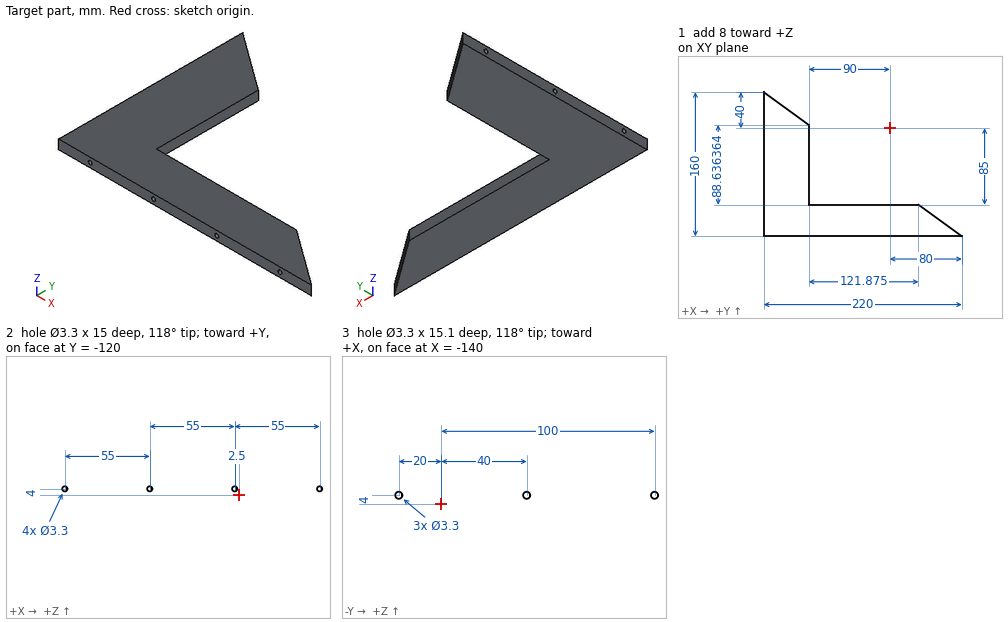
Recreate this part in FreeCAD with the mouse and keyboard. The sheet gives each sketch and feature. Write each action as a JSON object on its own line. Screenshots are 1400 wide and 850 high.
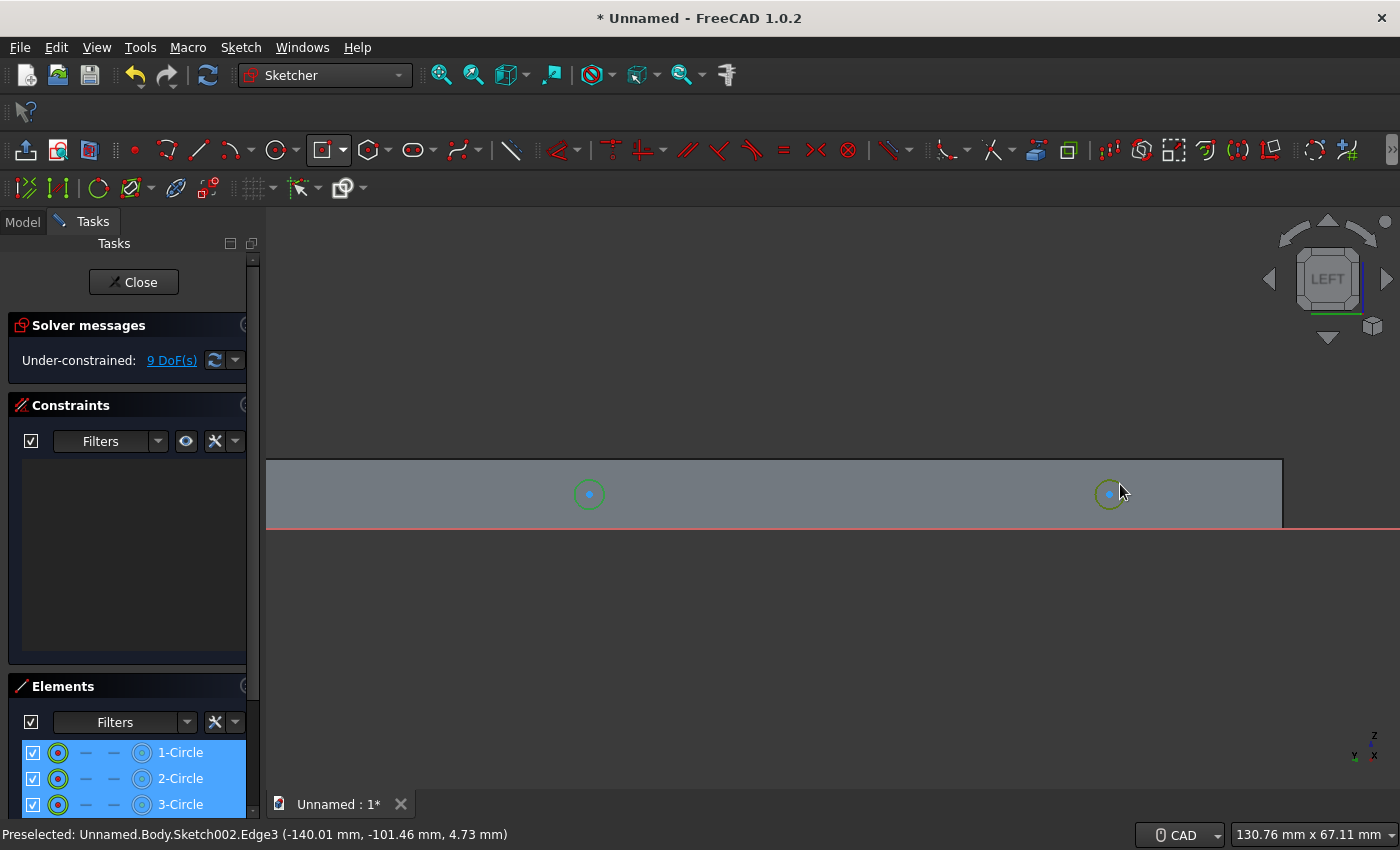
{"action": "key", "text": "e"}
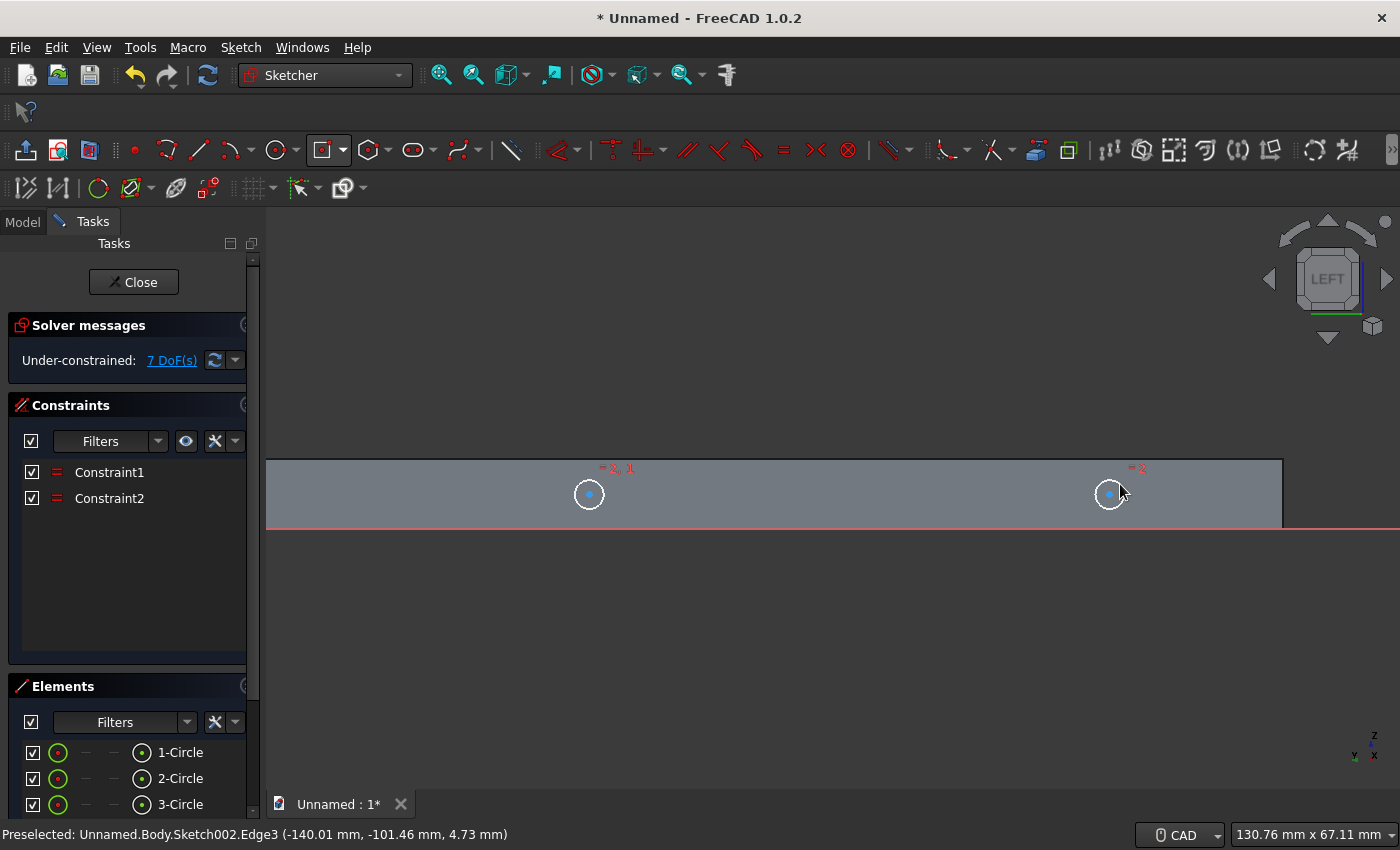
{"action": "scroll", "coordinate": [1120, 485], "scroll_direction": "down", "scroll_amount": 2}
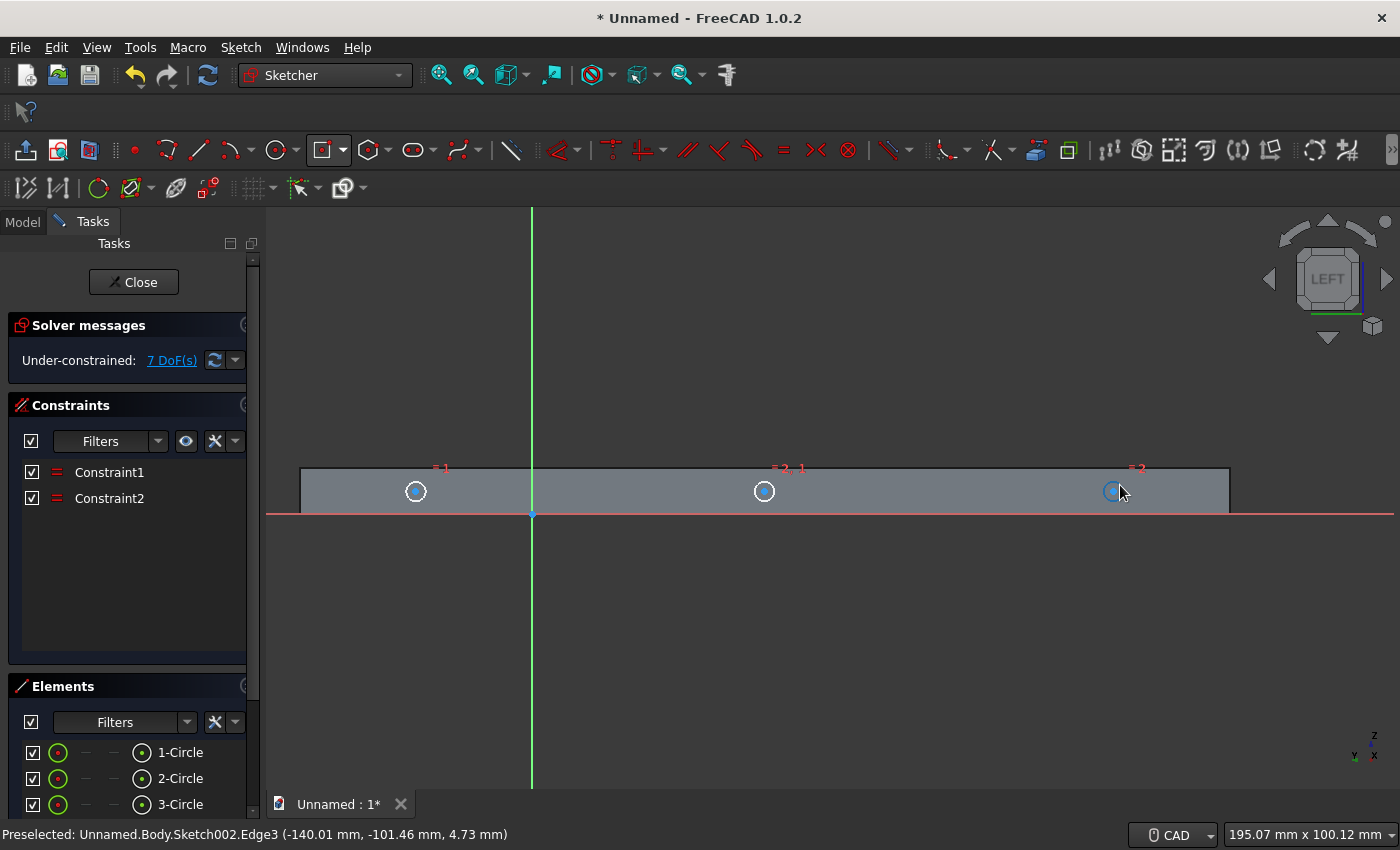
{"action": "left_click", "coordinate": [416, 492]}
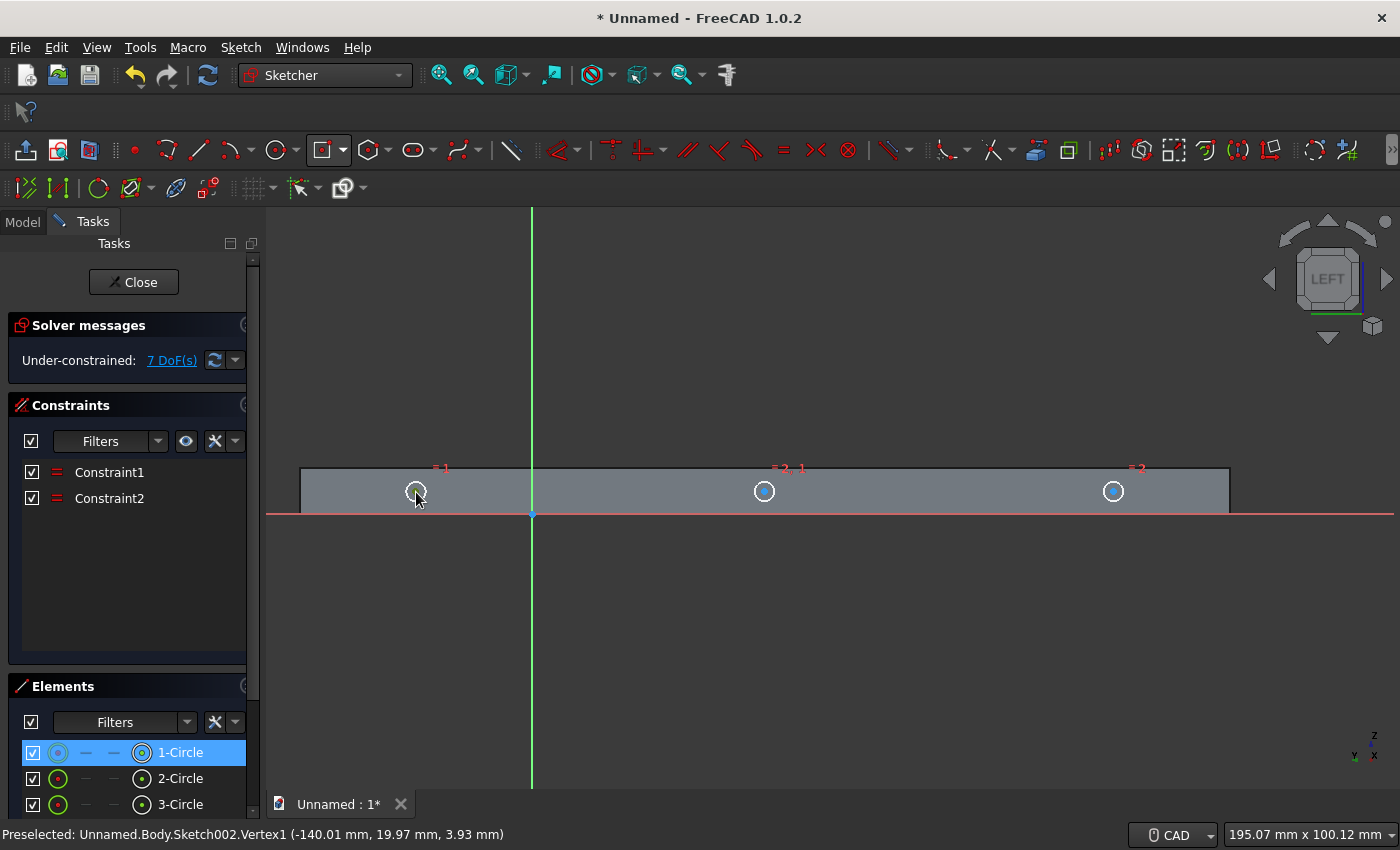
{"action": "left_click", "coordinate": [765, 492]}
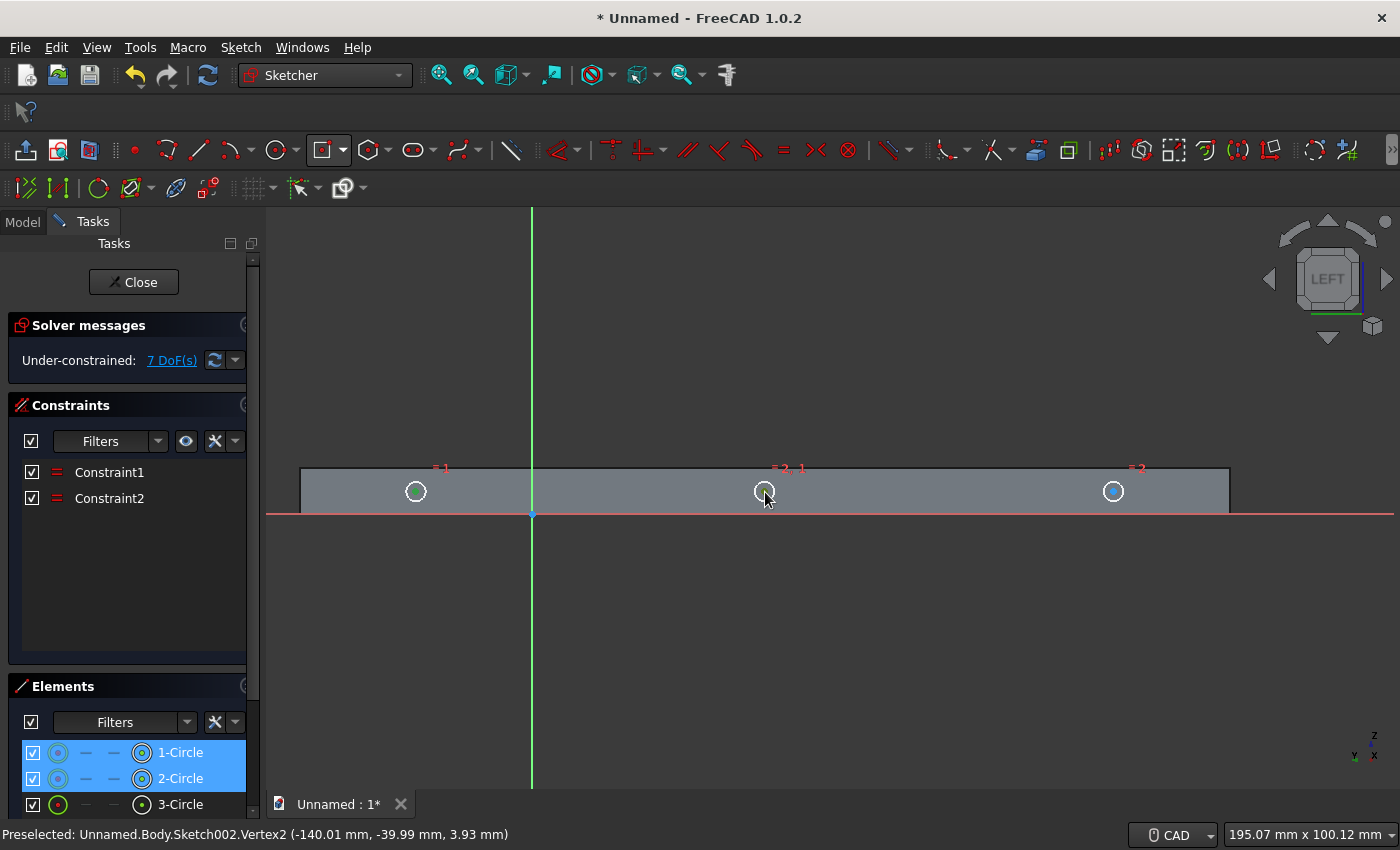
{"action": "left_click", "coordinate": [666, 150]}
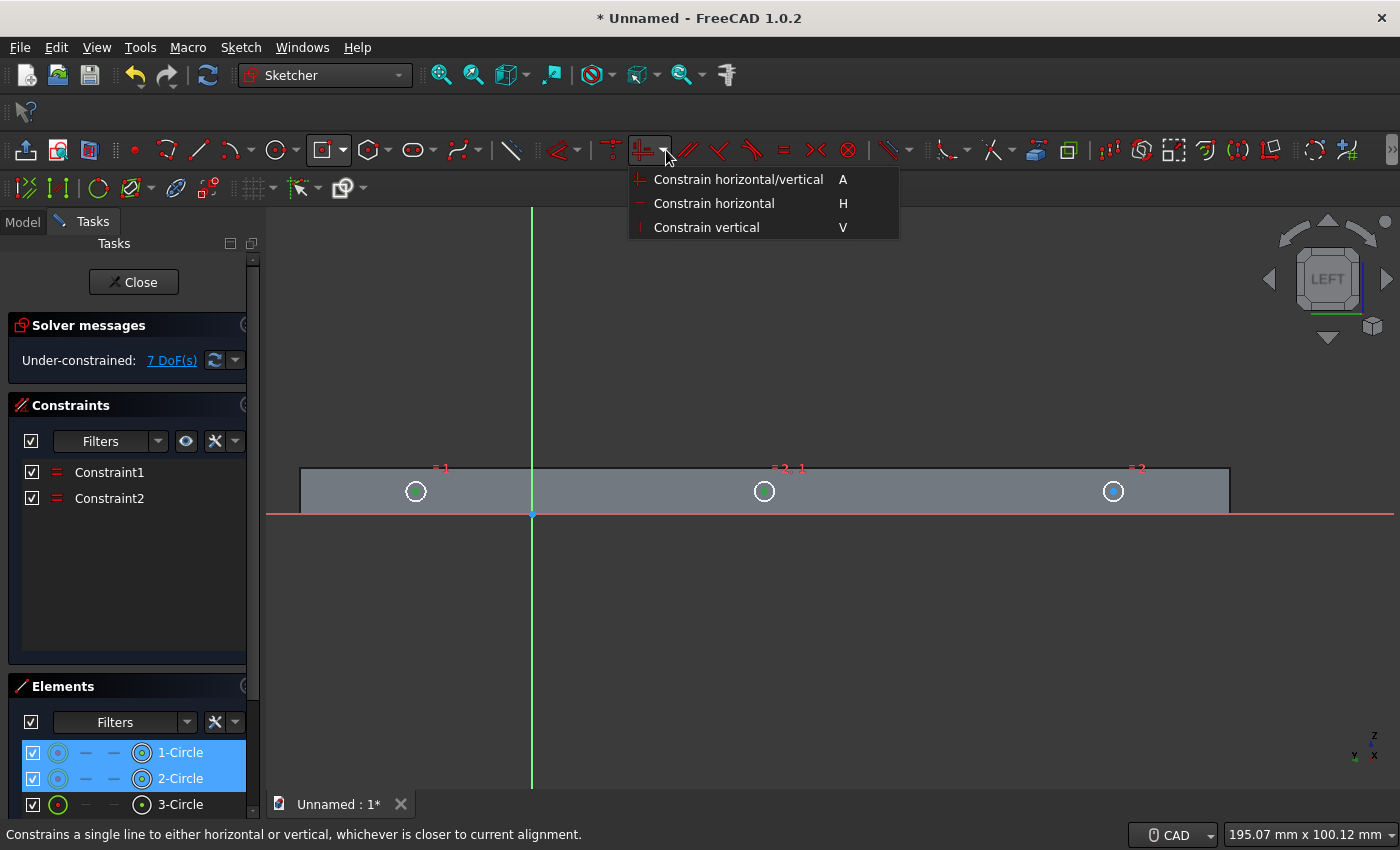
{"action": "left_click", "coordinate": [764, 203]}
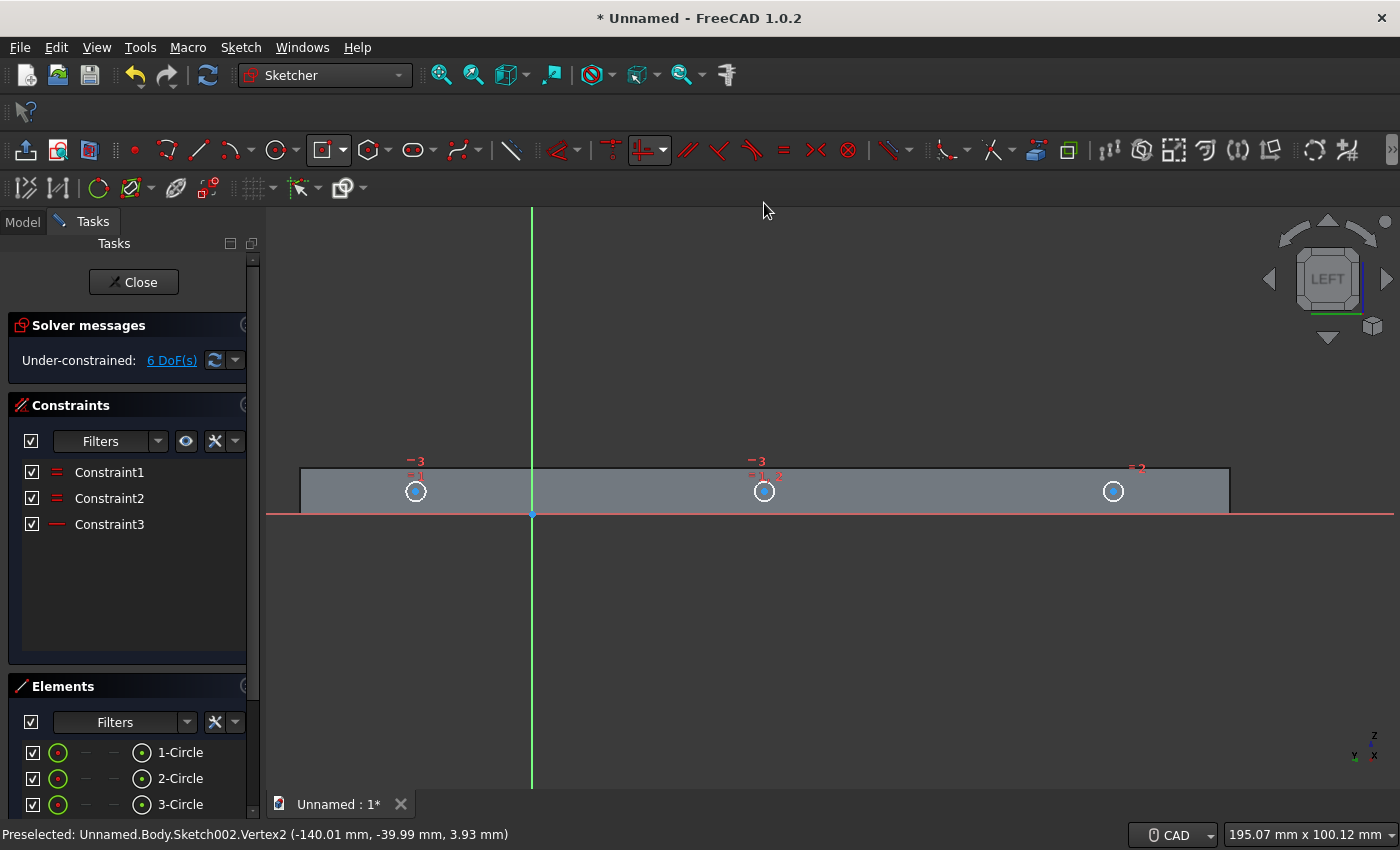
{"action": "left_click", "coordinate": [765, 492]}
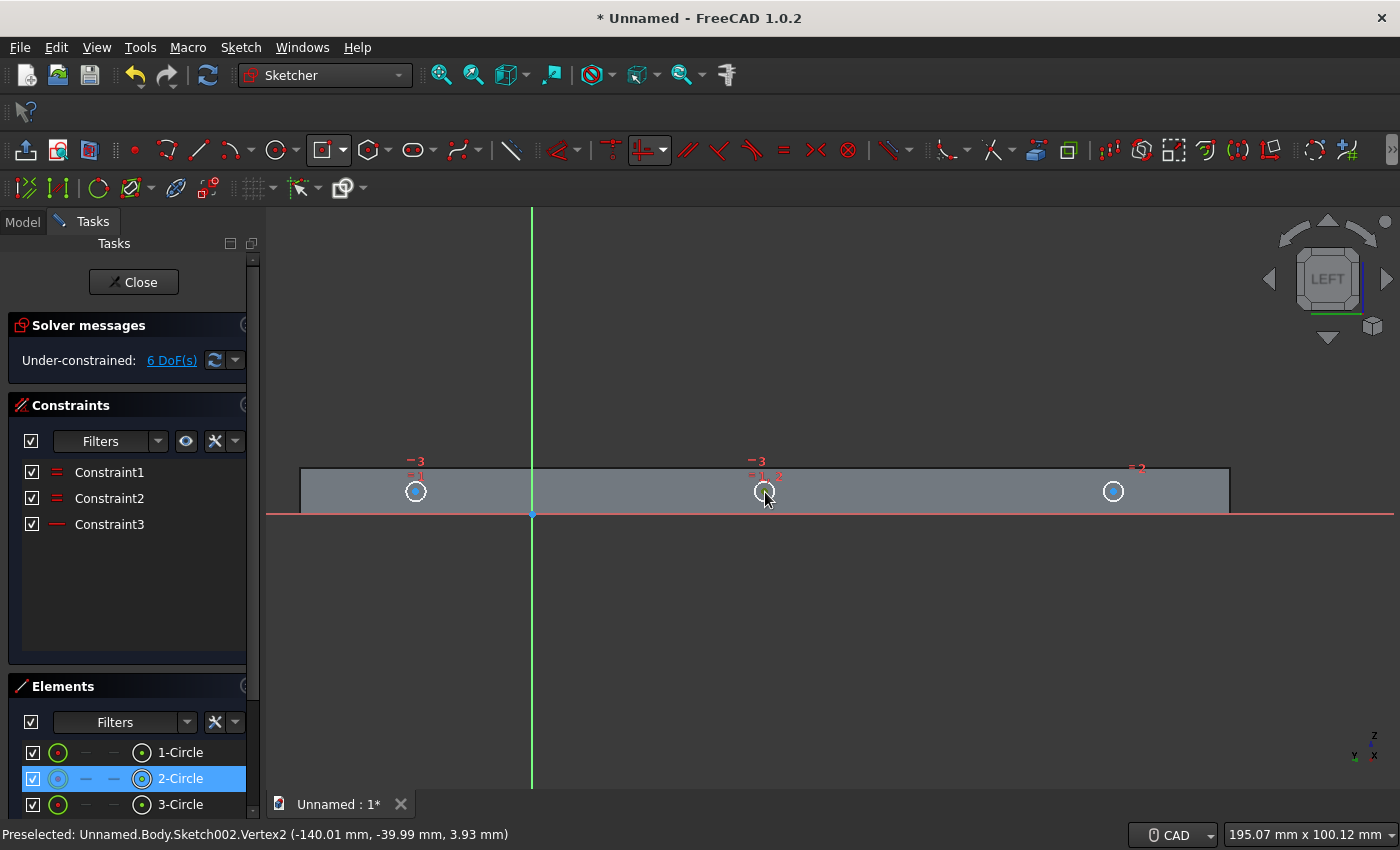
{"action": "left_click", "coordinate": [1113, 492]}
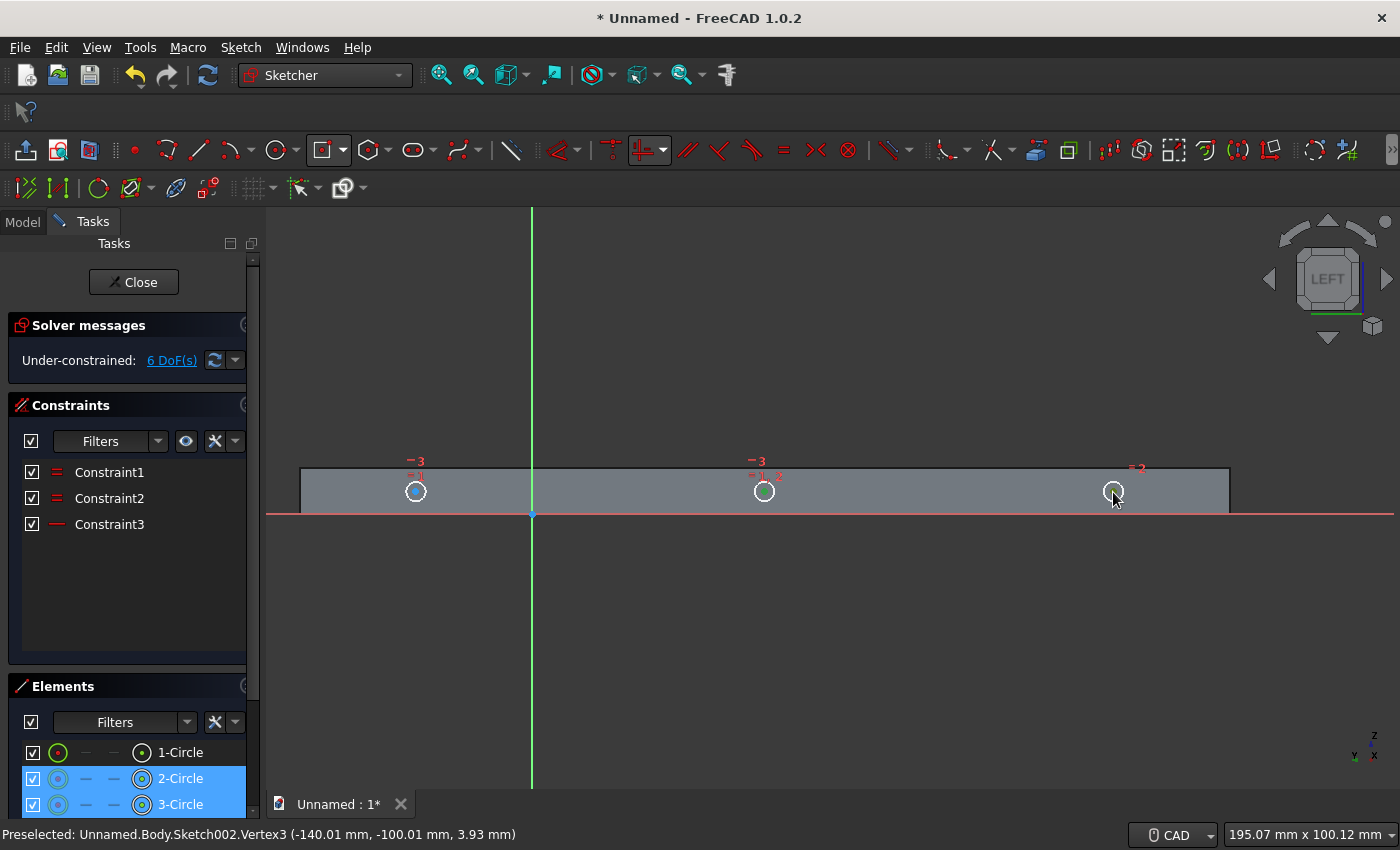
{"action": "key", "text": "h"}